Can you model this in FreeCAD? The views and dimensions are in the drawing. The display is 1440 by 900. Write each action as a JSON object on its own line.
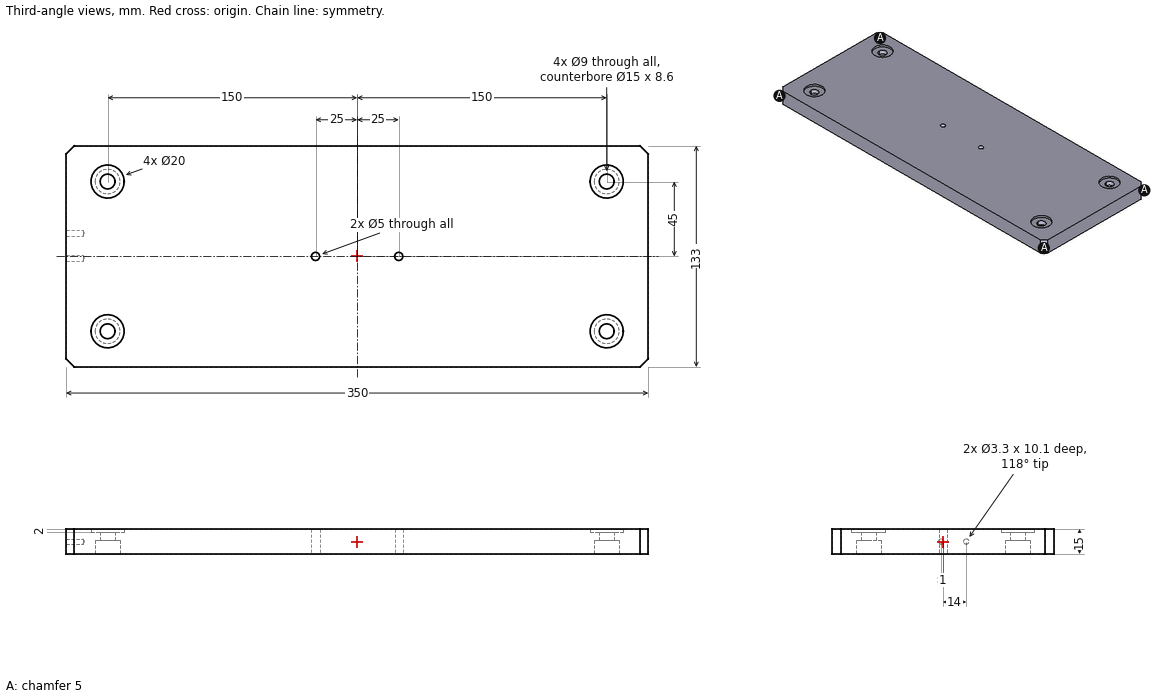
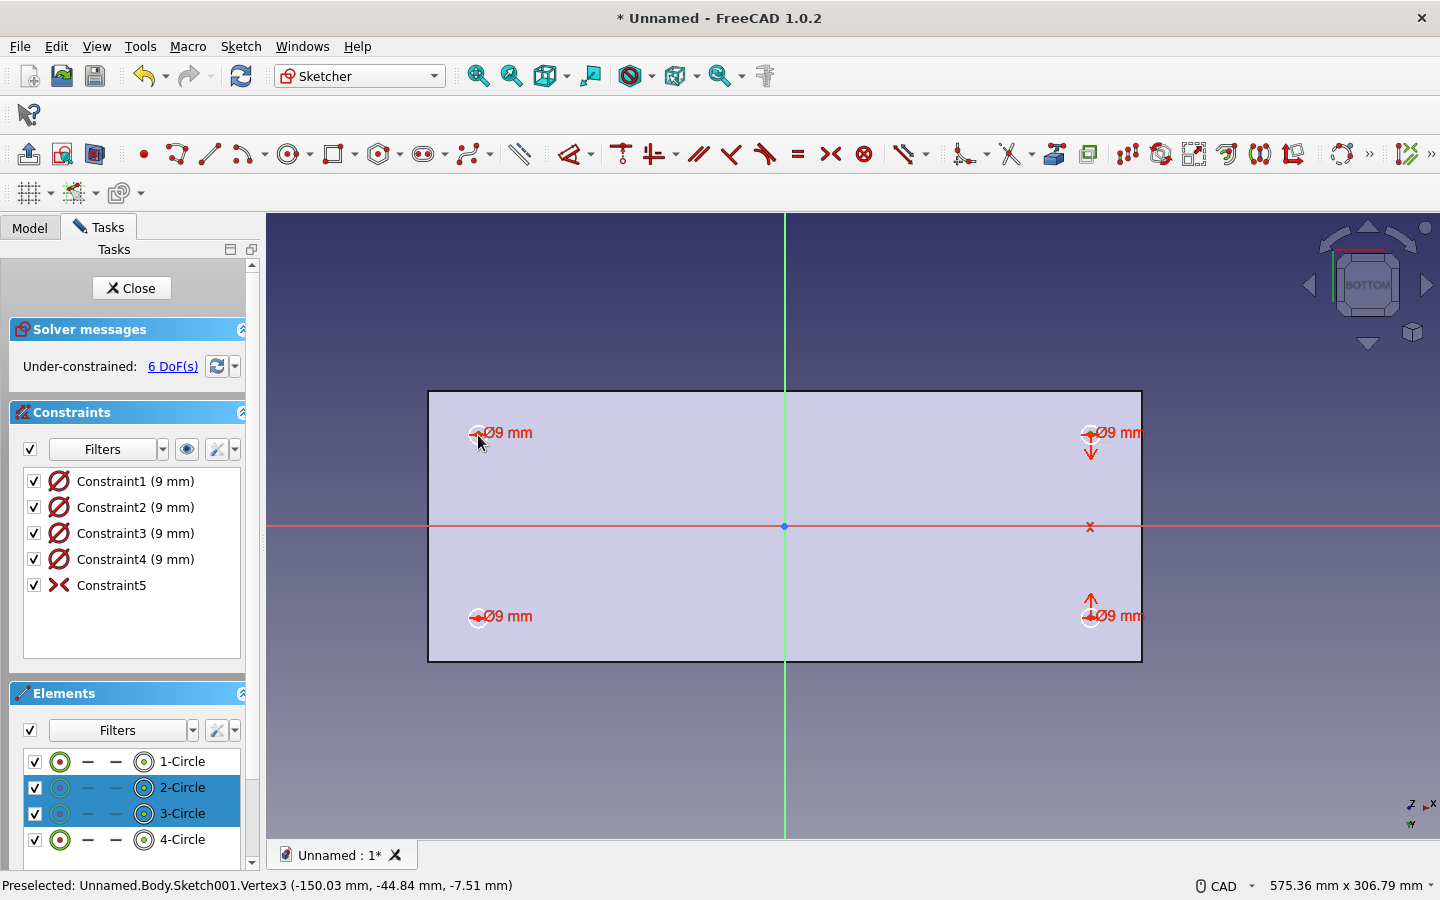
{"action": "left_click", "coordinate": [785, 770]}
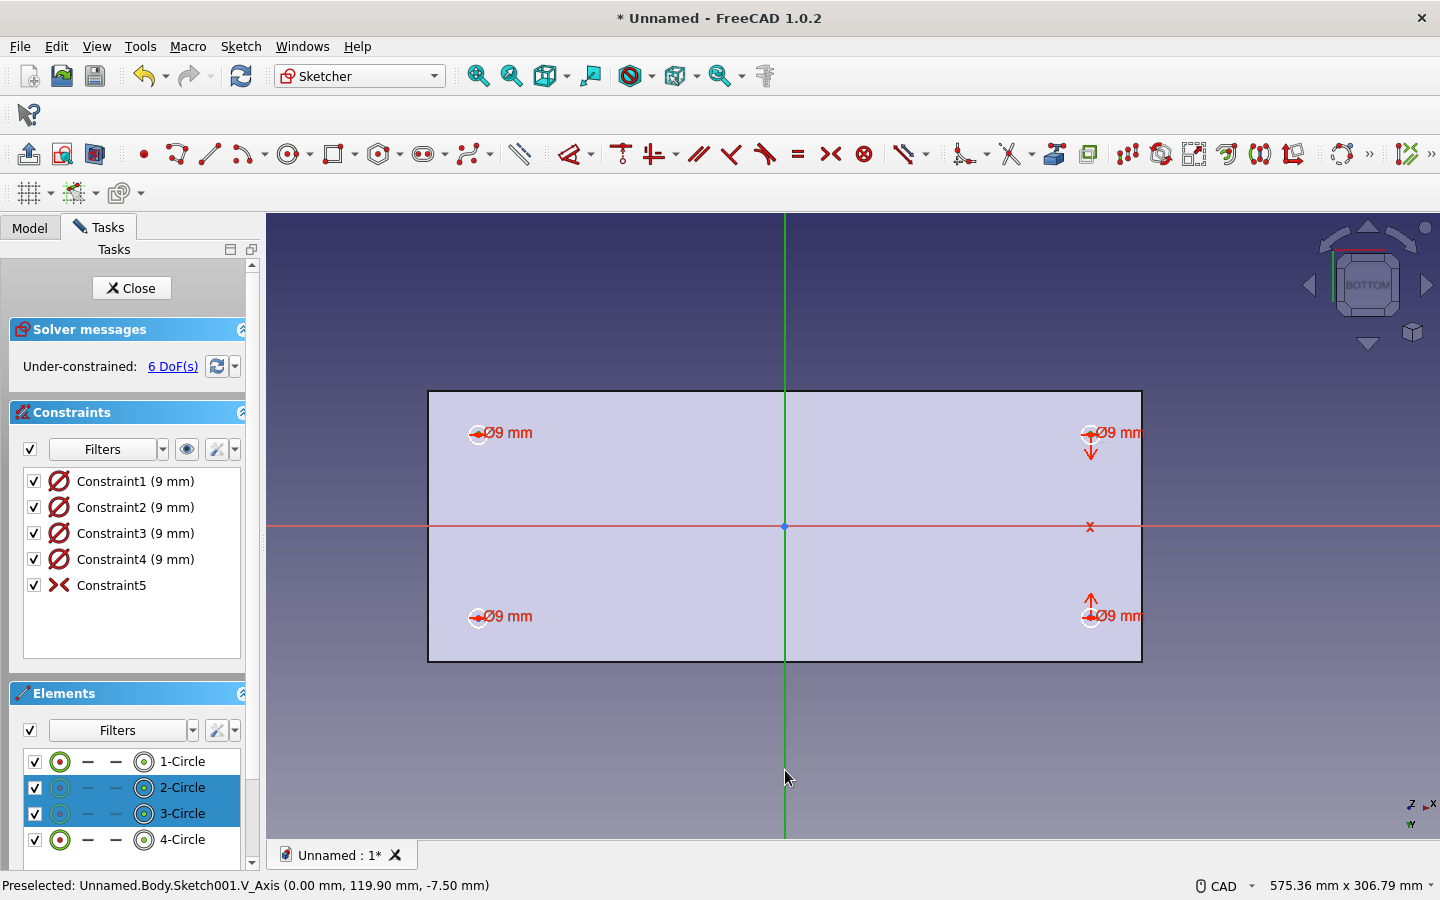
{"action": "key", "text": "s"}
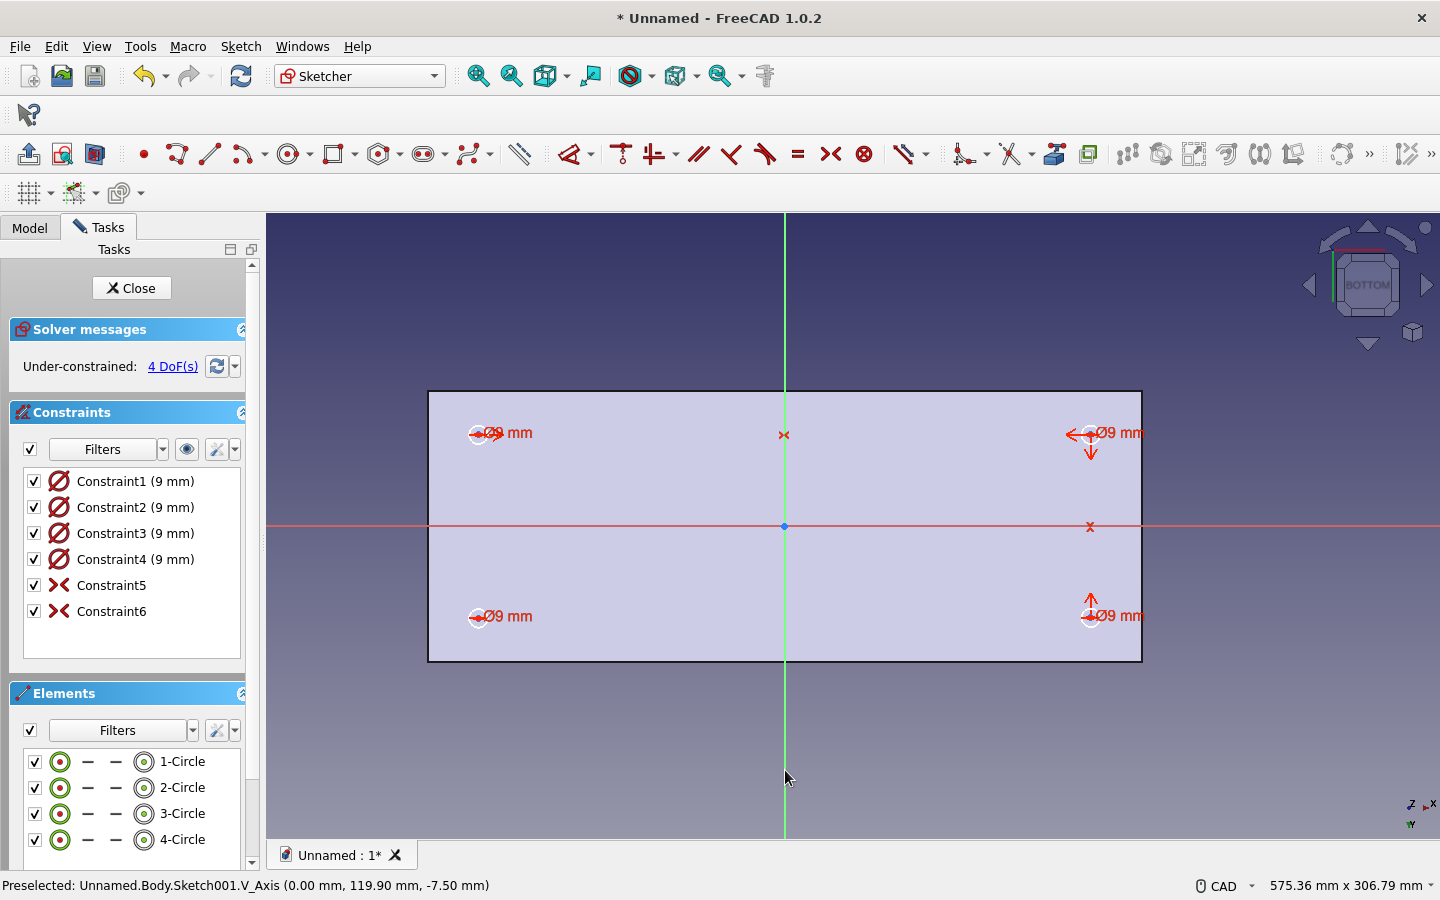
{"action": "left_click", "coordinate": [1091, 618]}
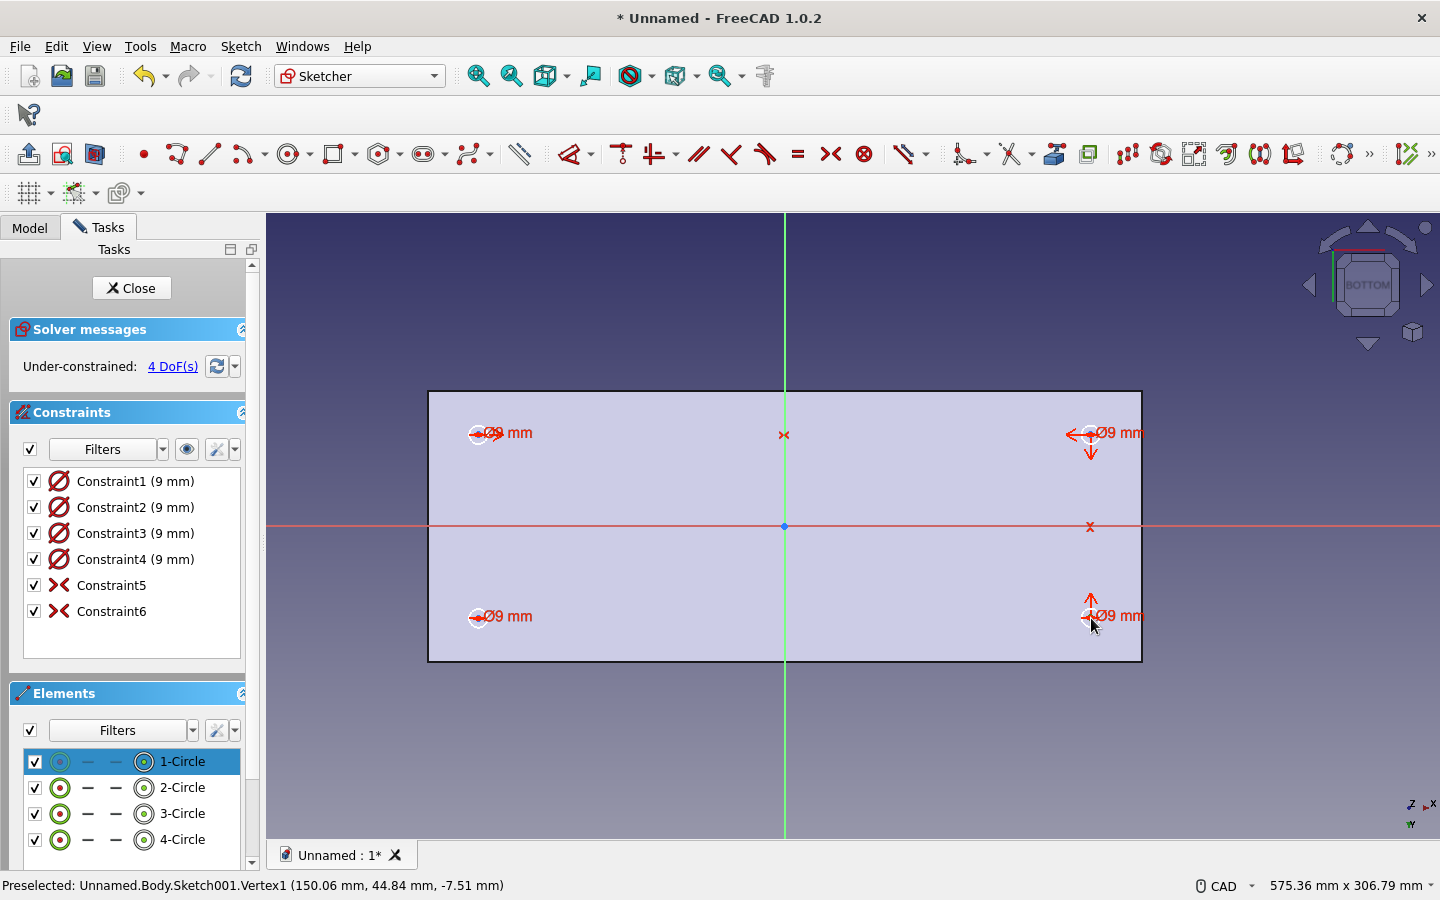
{"action": "left_click", "coordinate": [478, 618]}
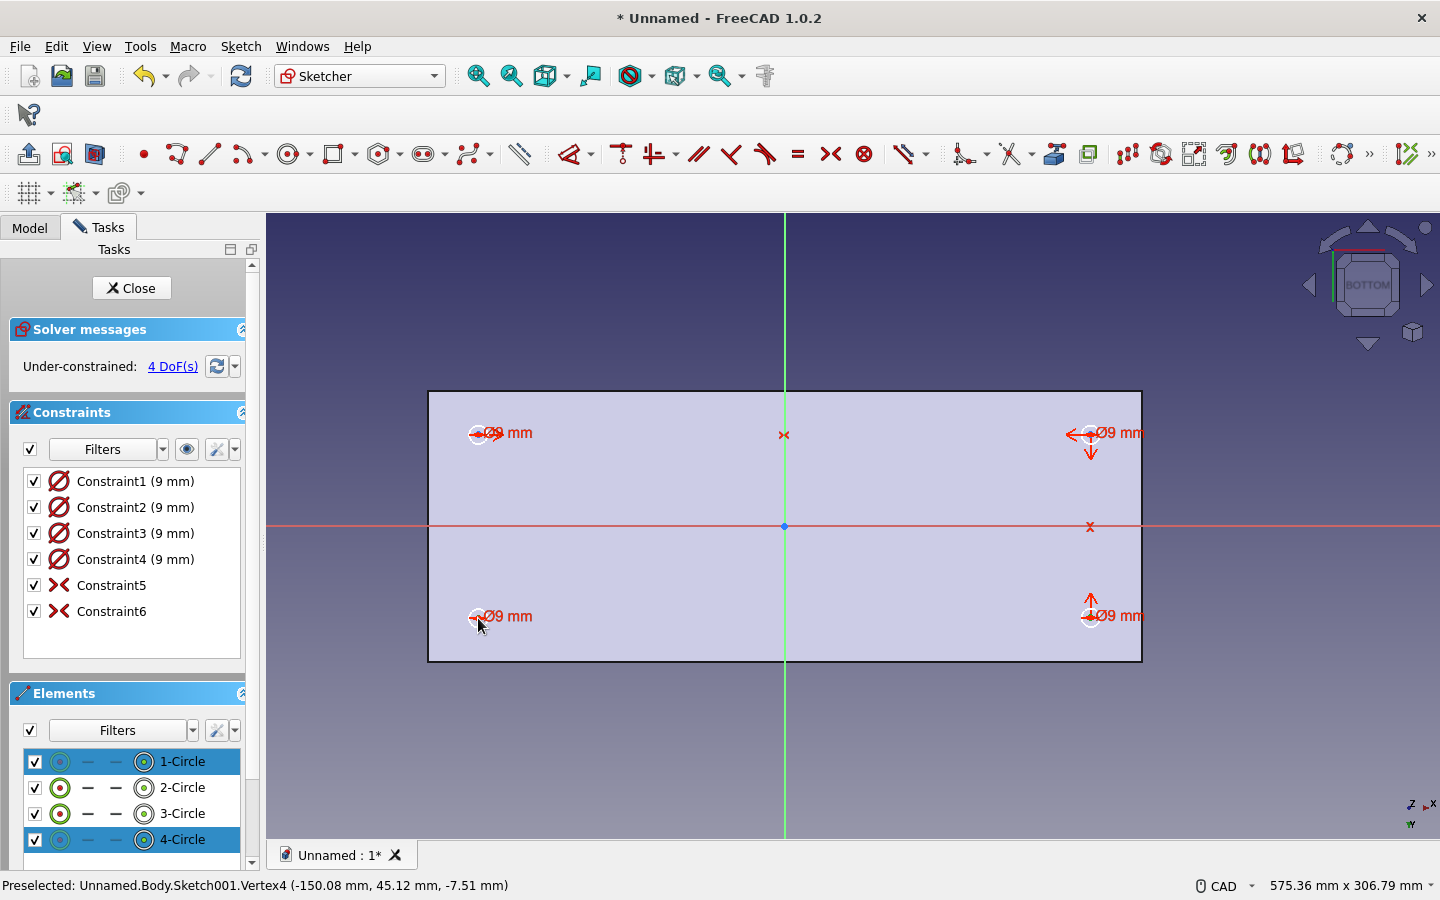
{"action": "left_click", "coordinate": [785, 770]}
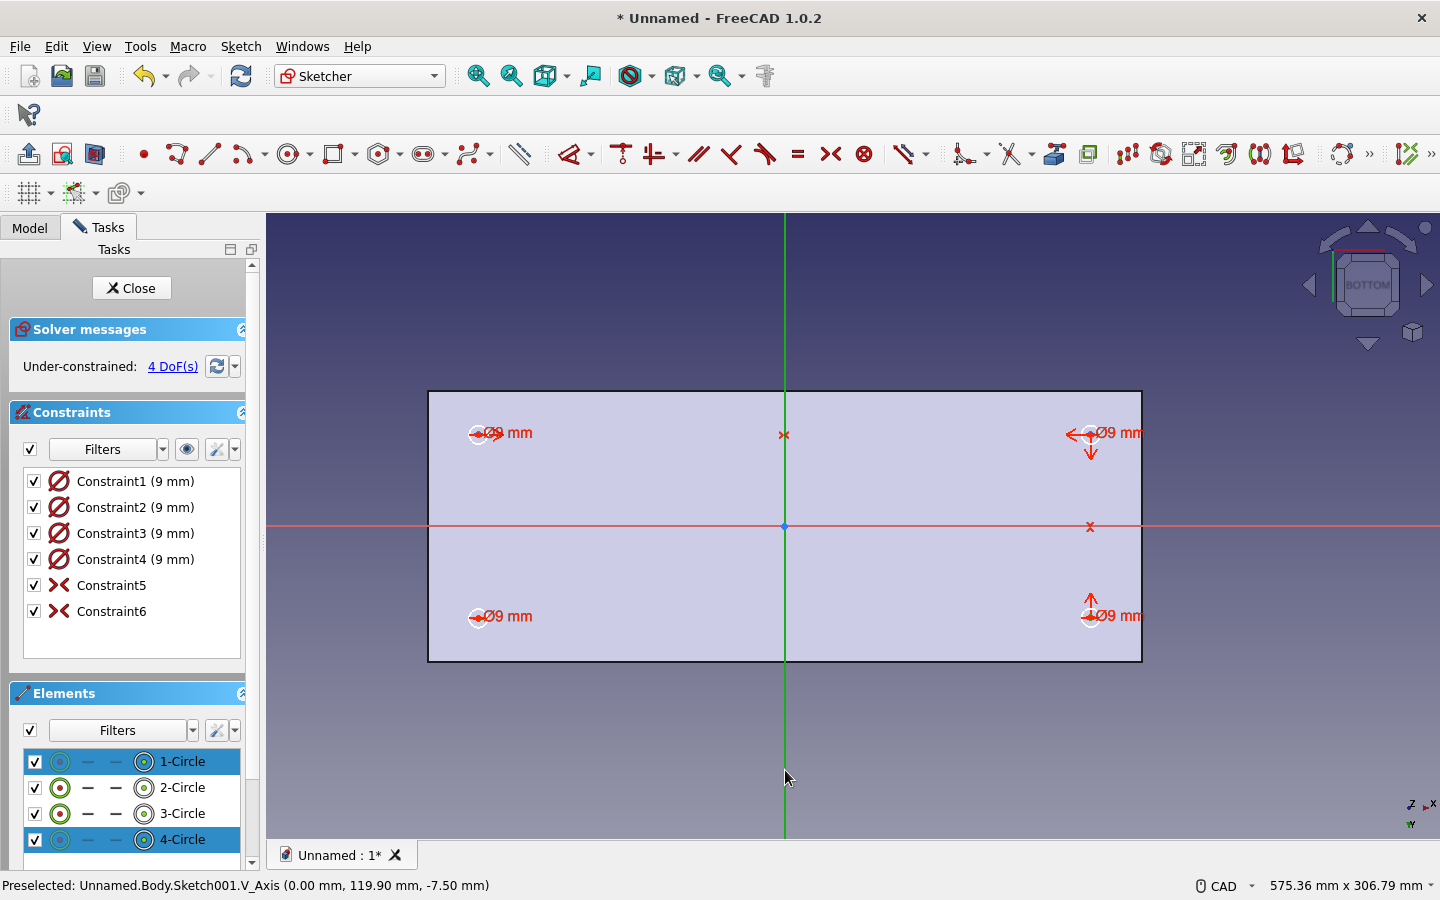
{"action": "key", "text": "s"}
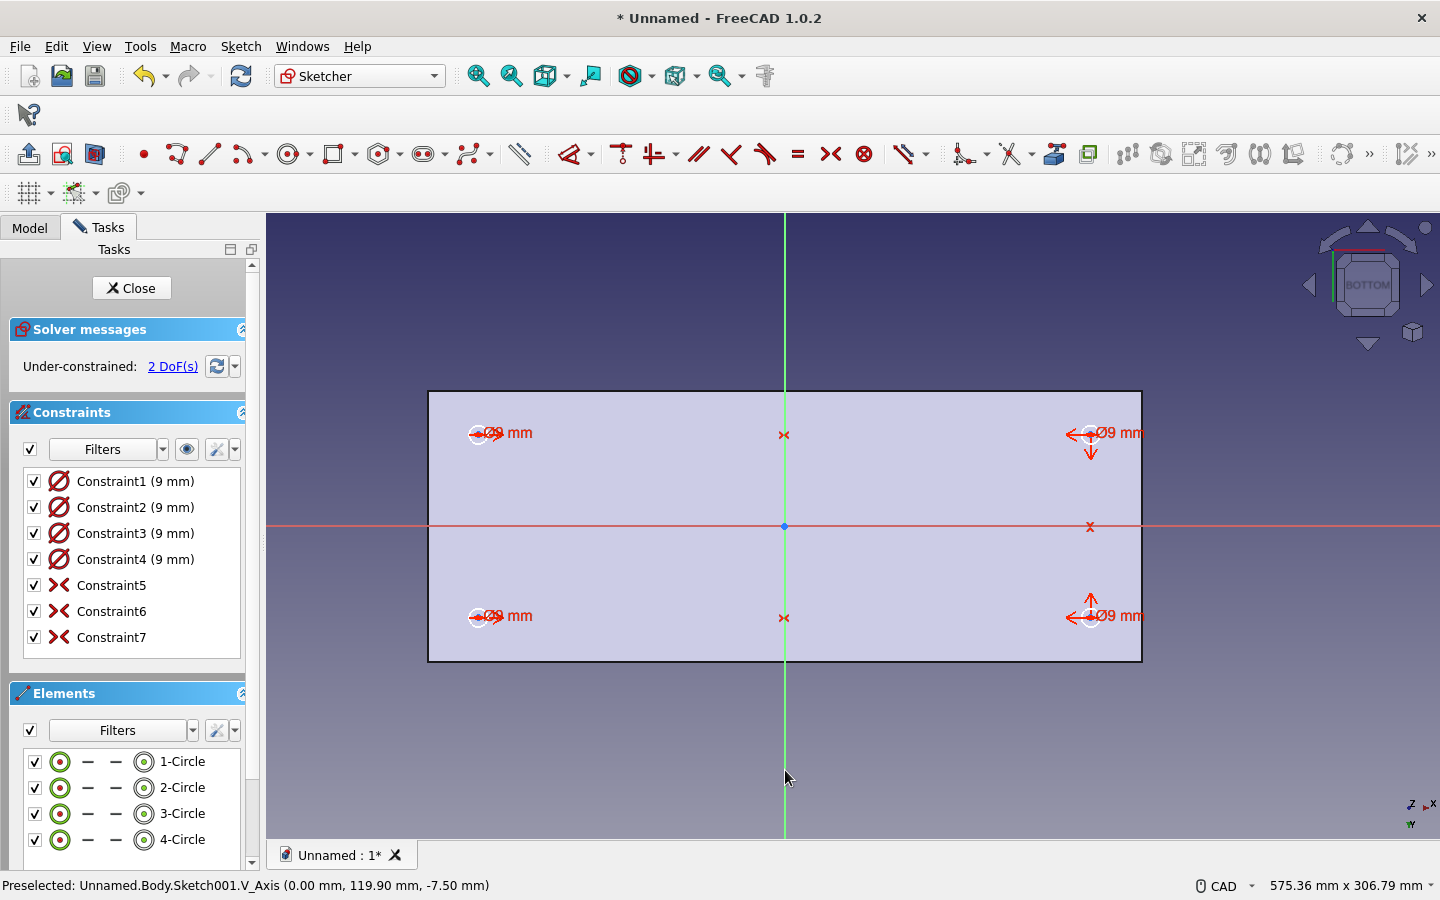
{"action": "key", "text": "d"}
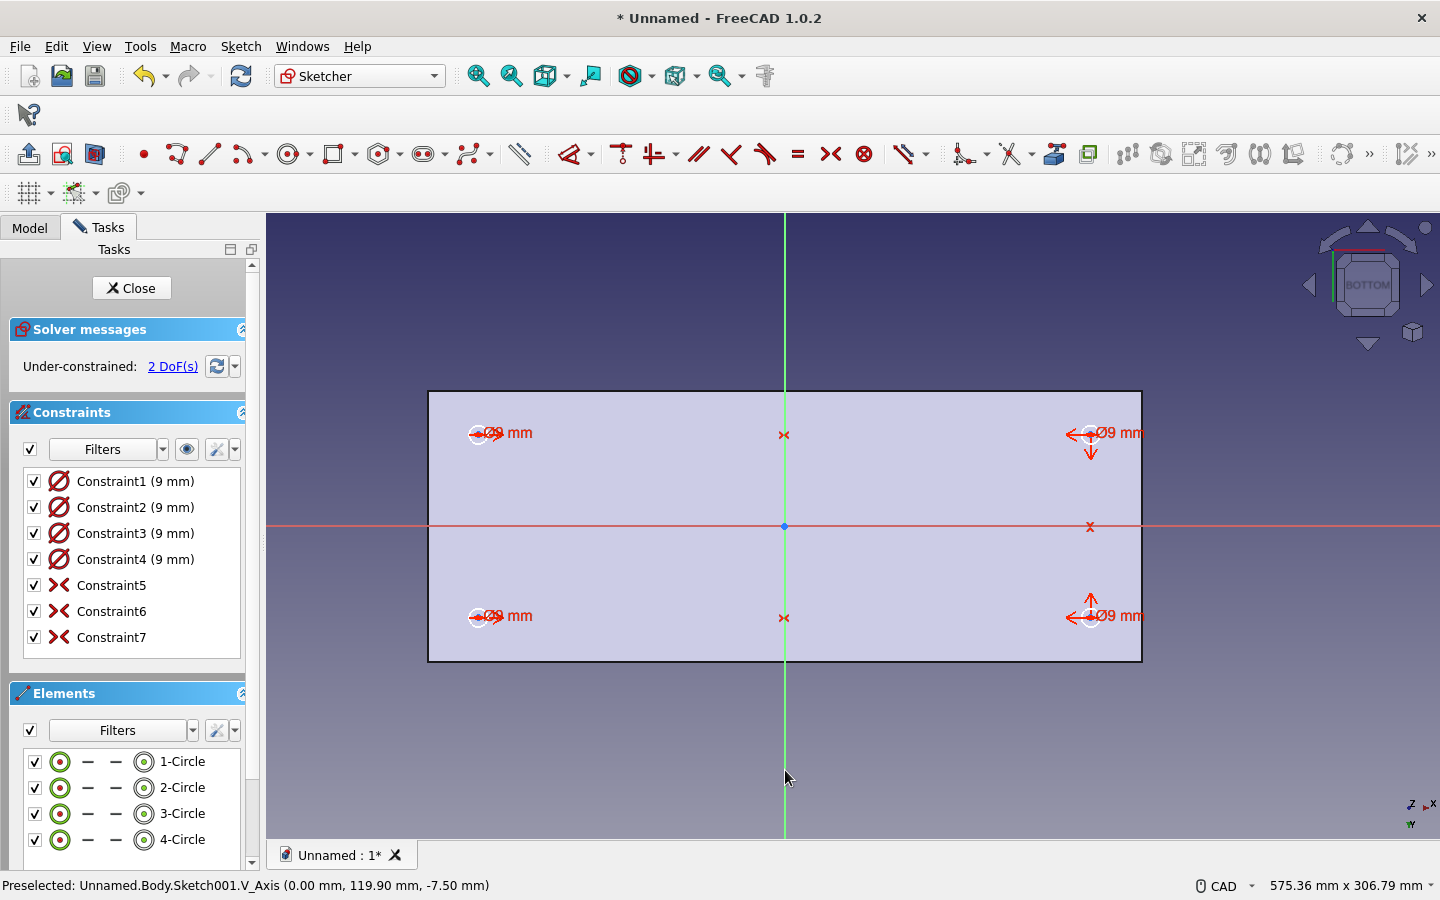
{"action": "left_click", "coordinate": [1091, 618]}
{"action": "left_click", "coordinate": [1125, 572]}